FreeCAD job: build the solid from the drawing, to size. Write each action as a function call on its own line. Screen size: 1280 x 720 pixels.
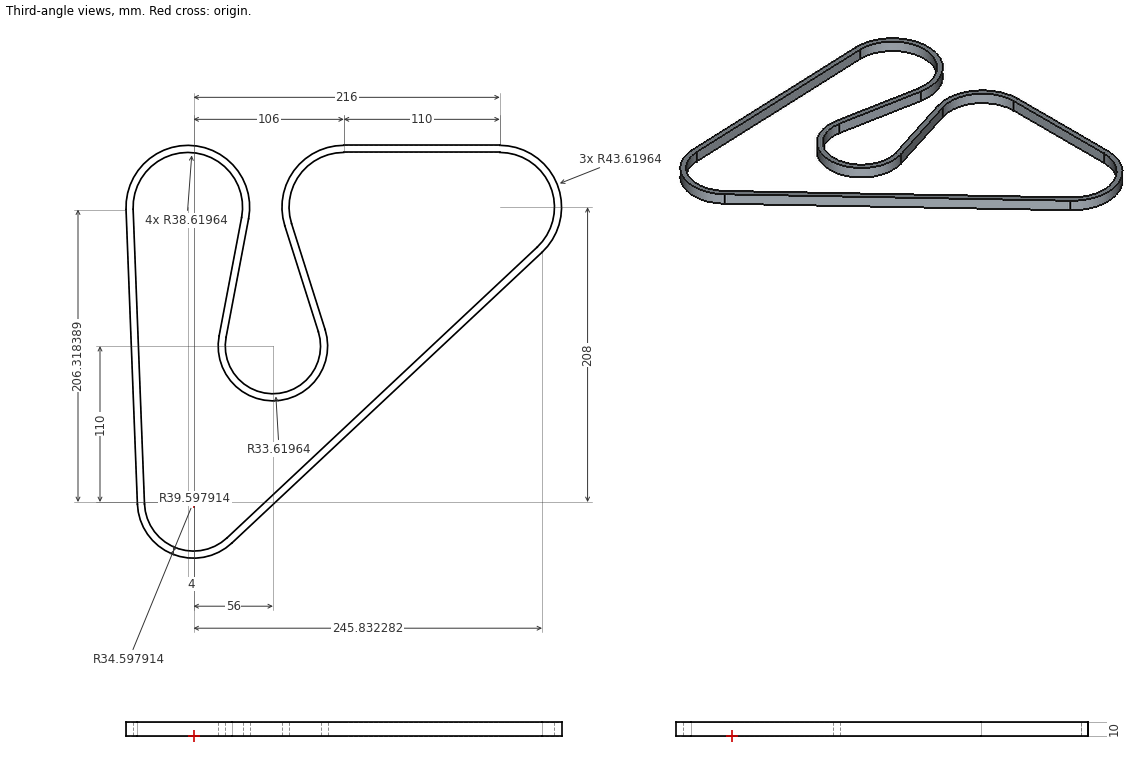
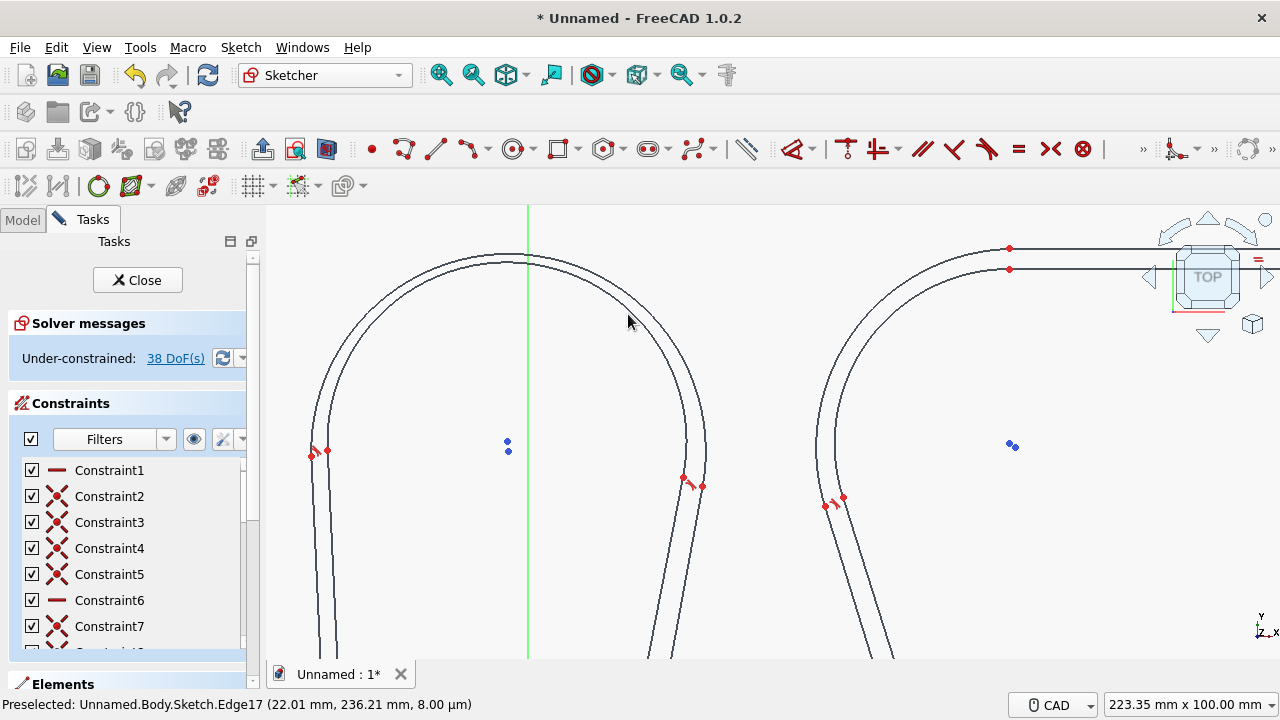
click(661, 591)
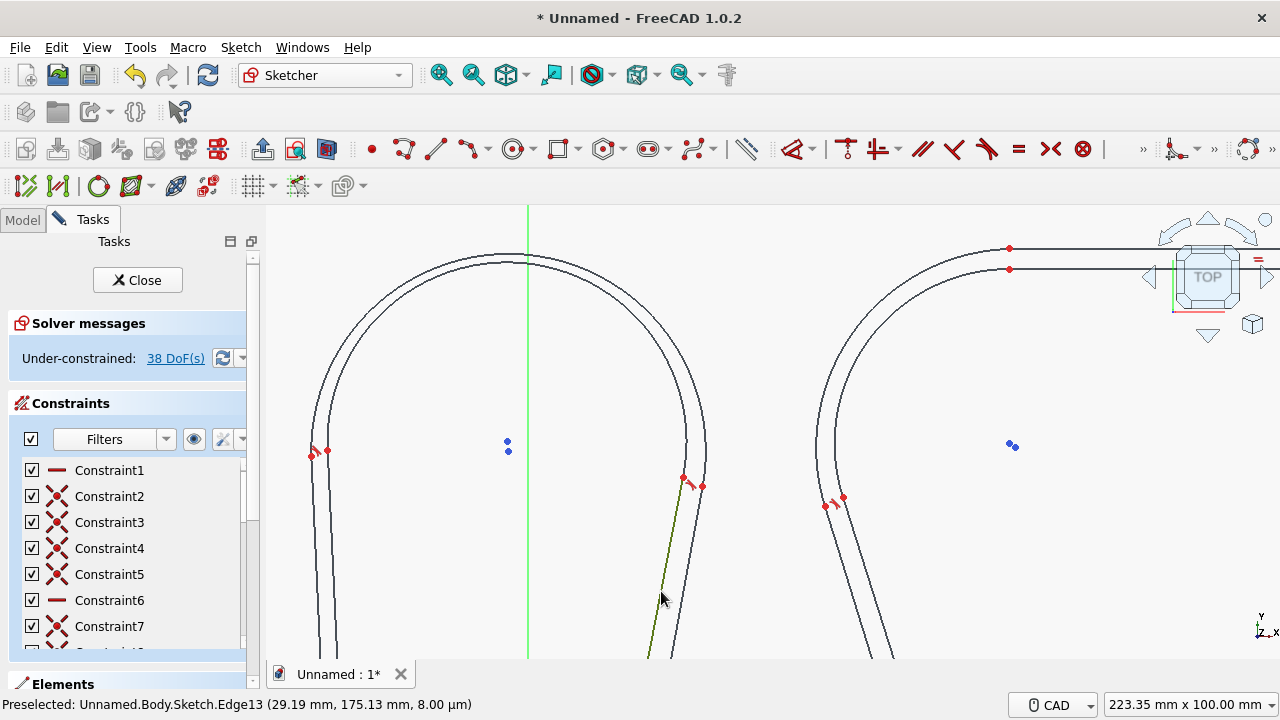
click(630, 311)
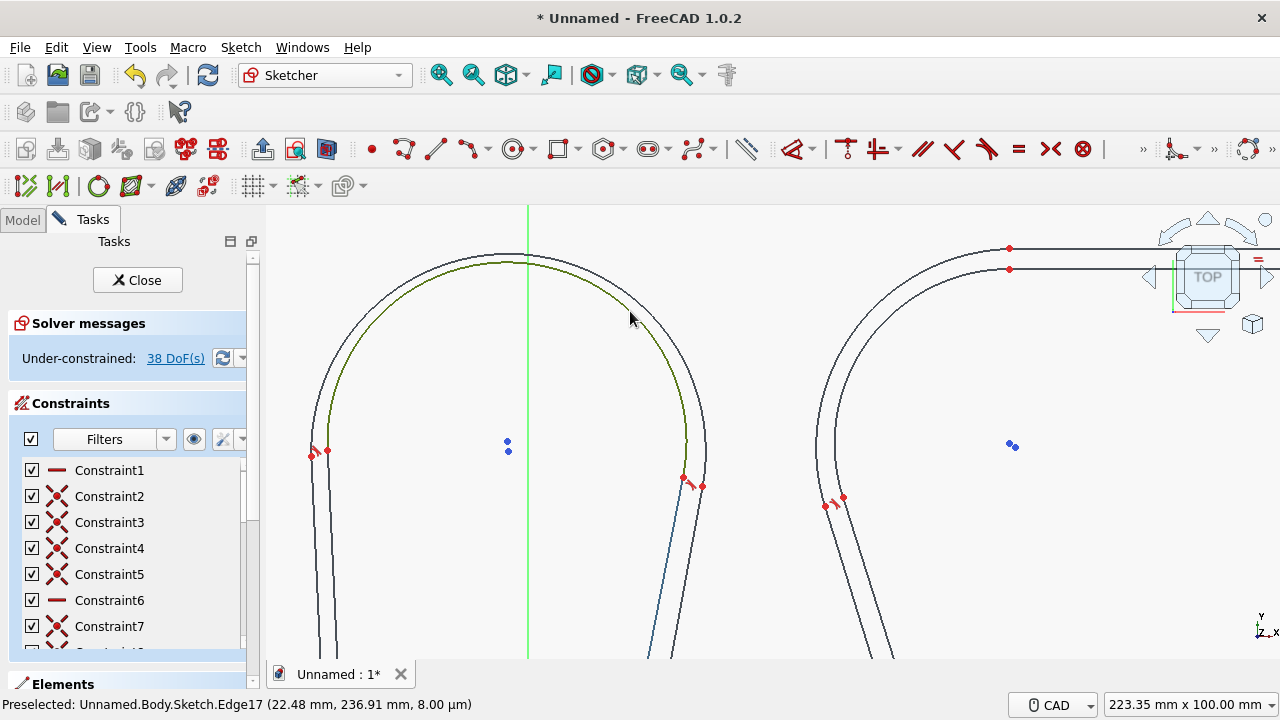
key(t)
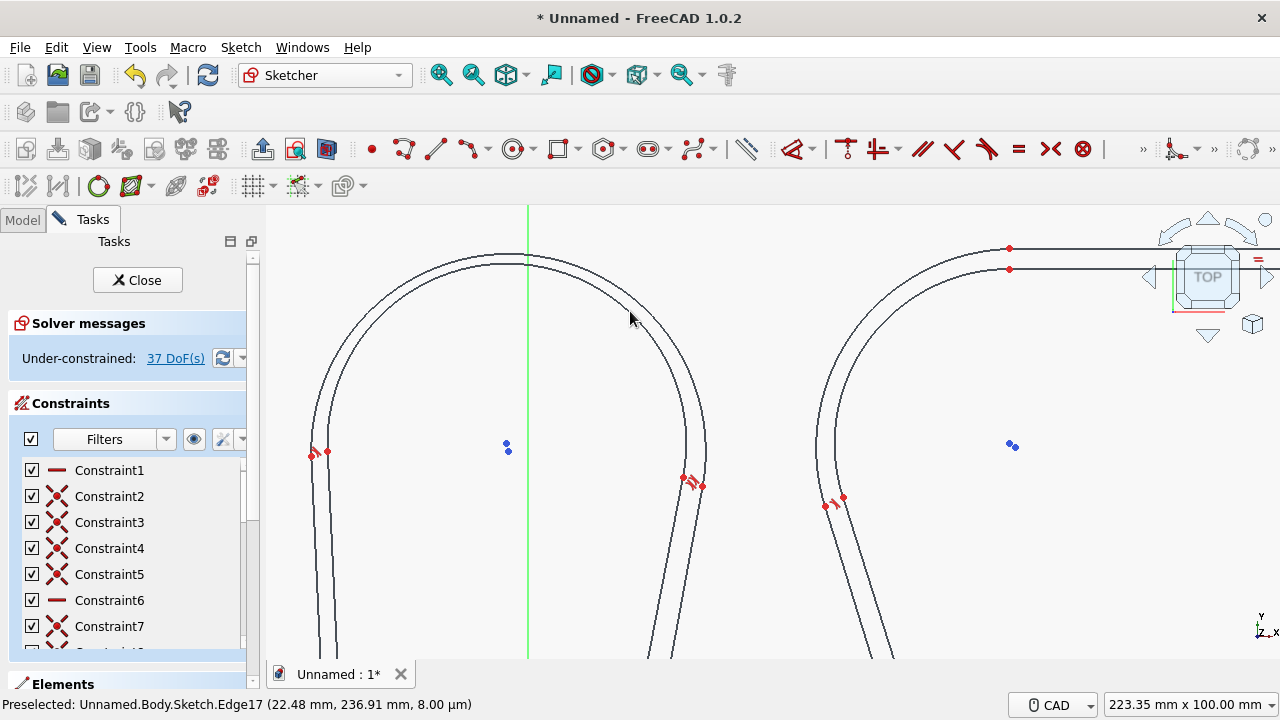
click(661, 591)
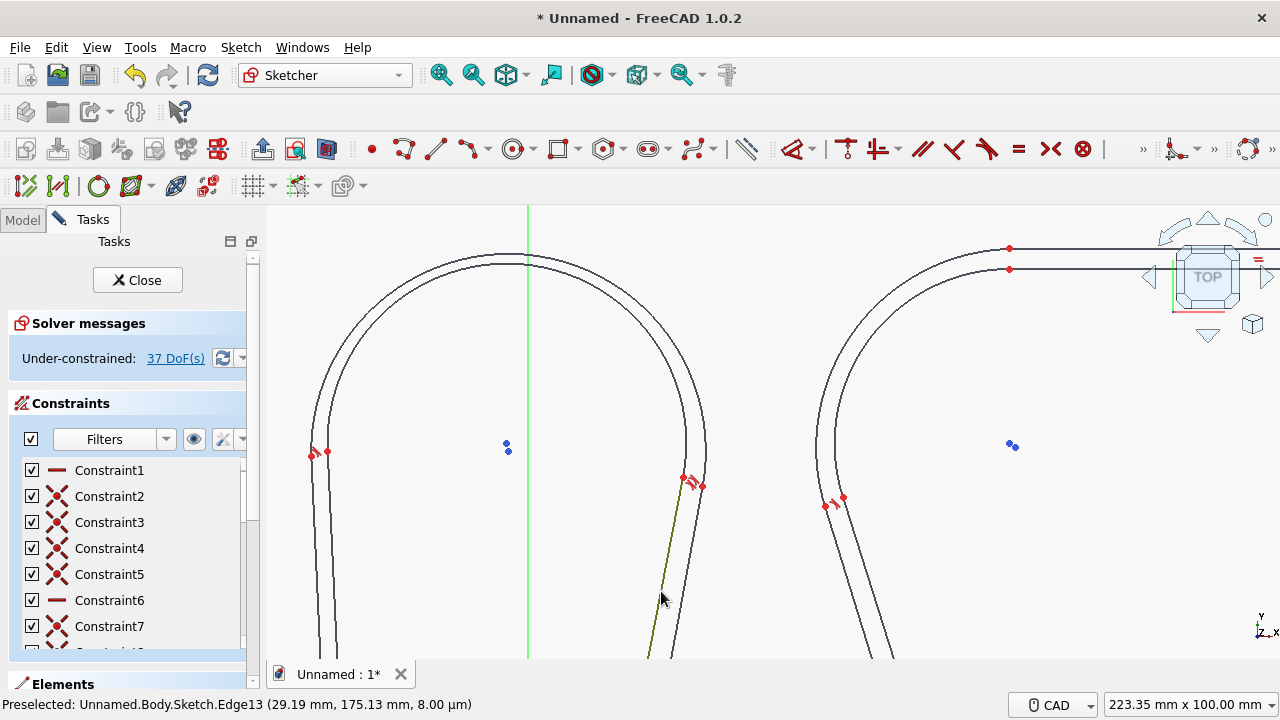
scroll(629, 314, down, 8)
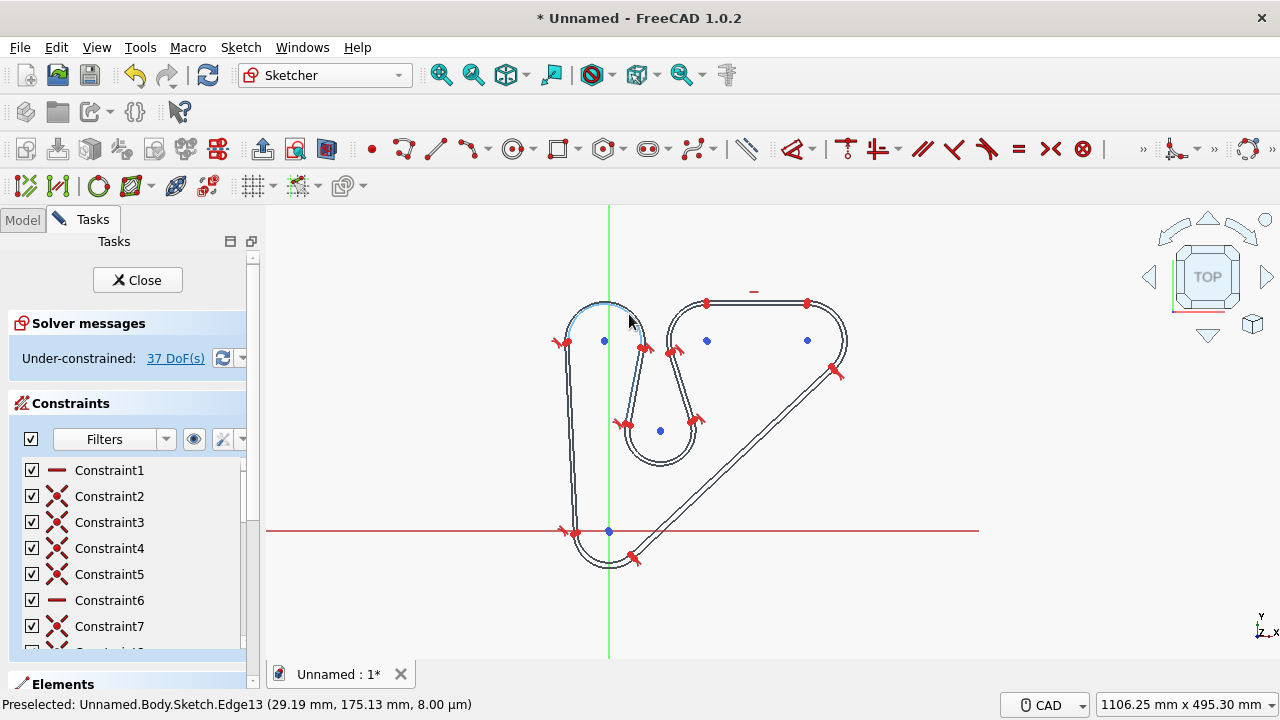
scroll(638, 458, up, 7)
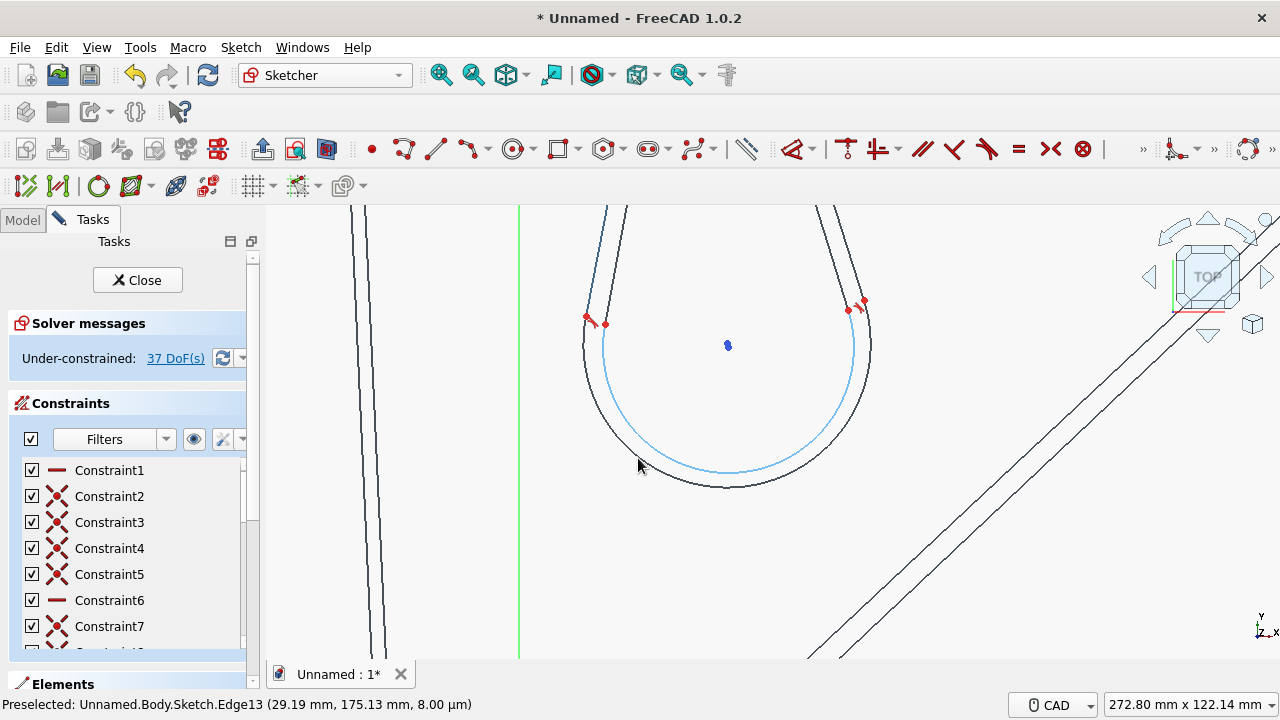
click(638, 457)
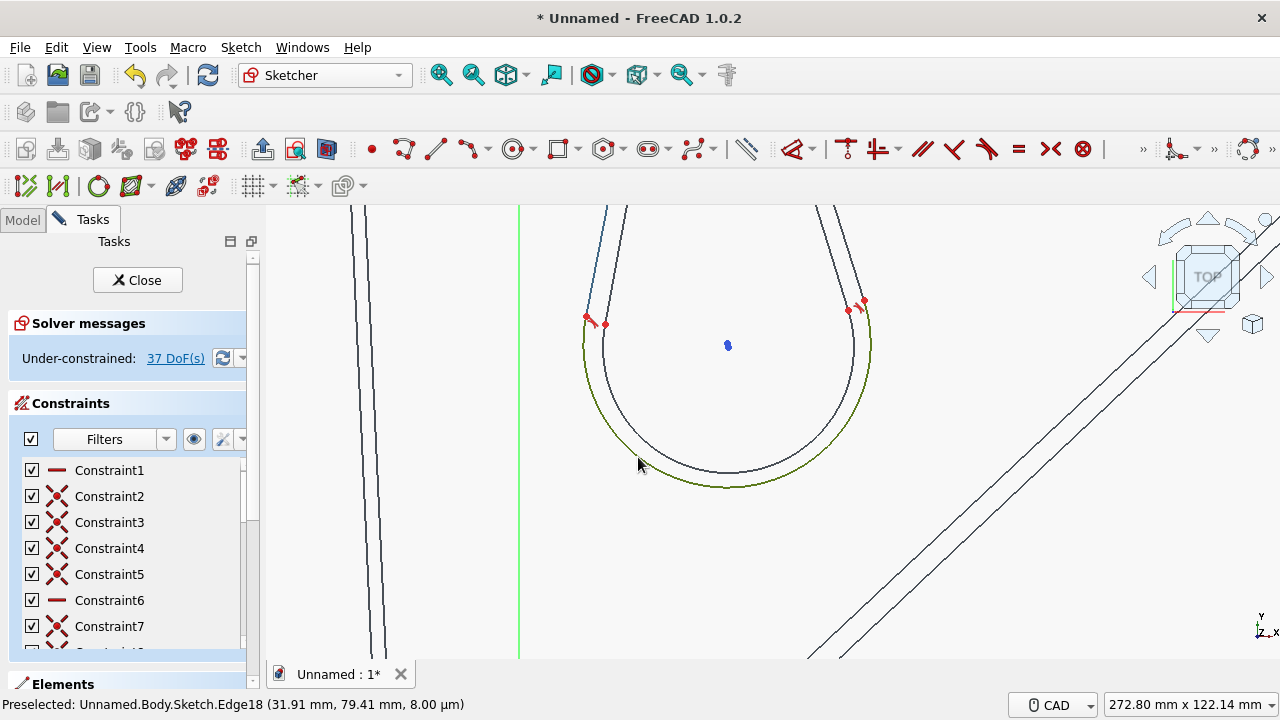
click(988, 150)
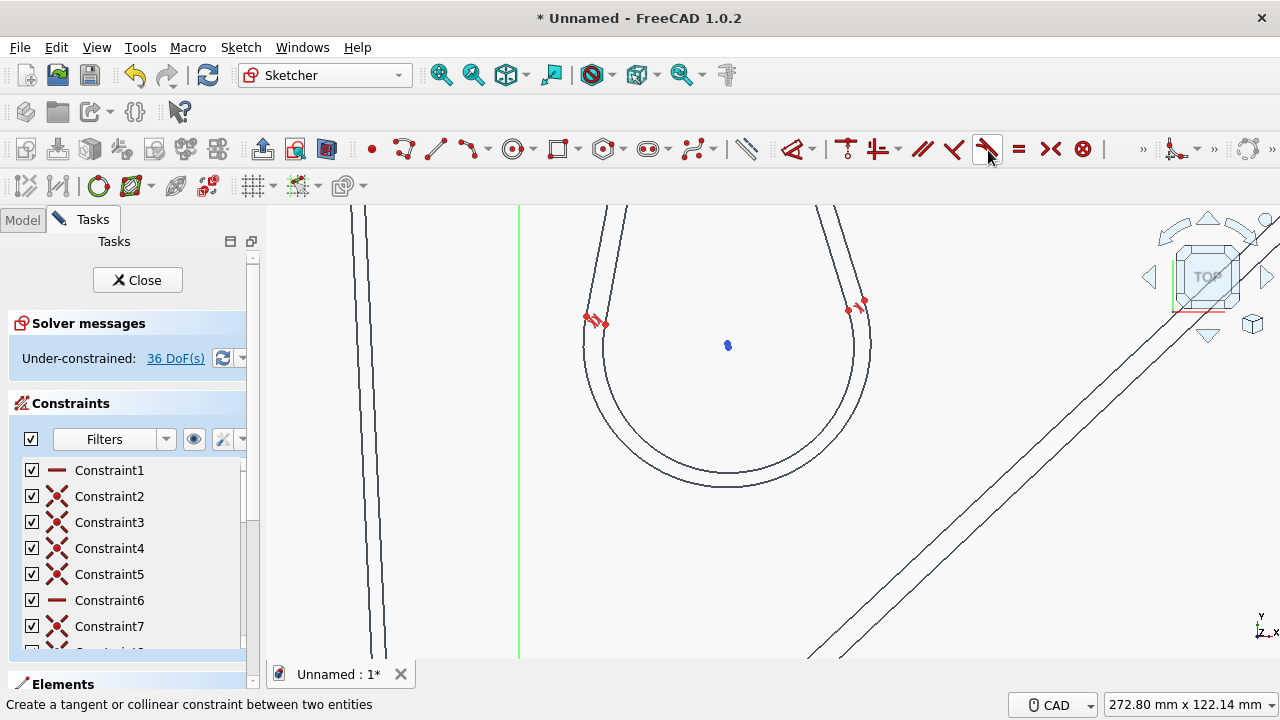
click(847, 245)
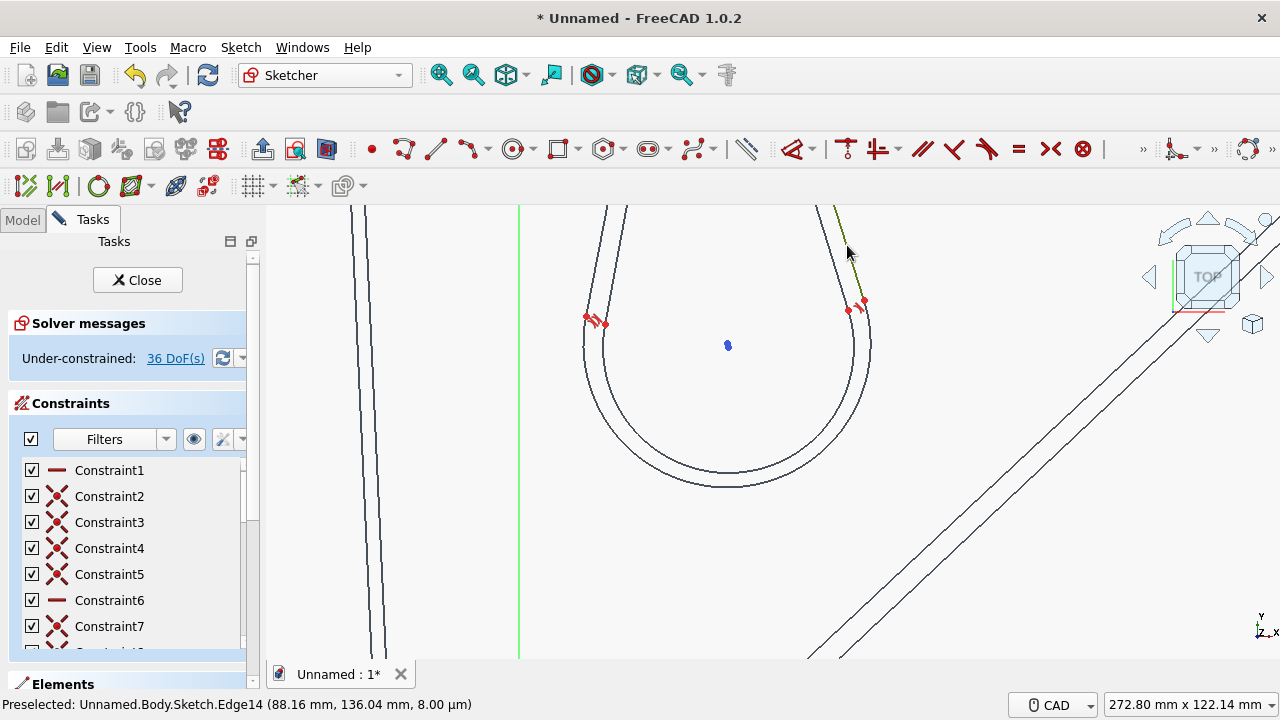
click(638, 456)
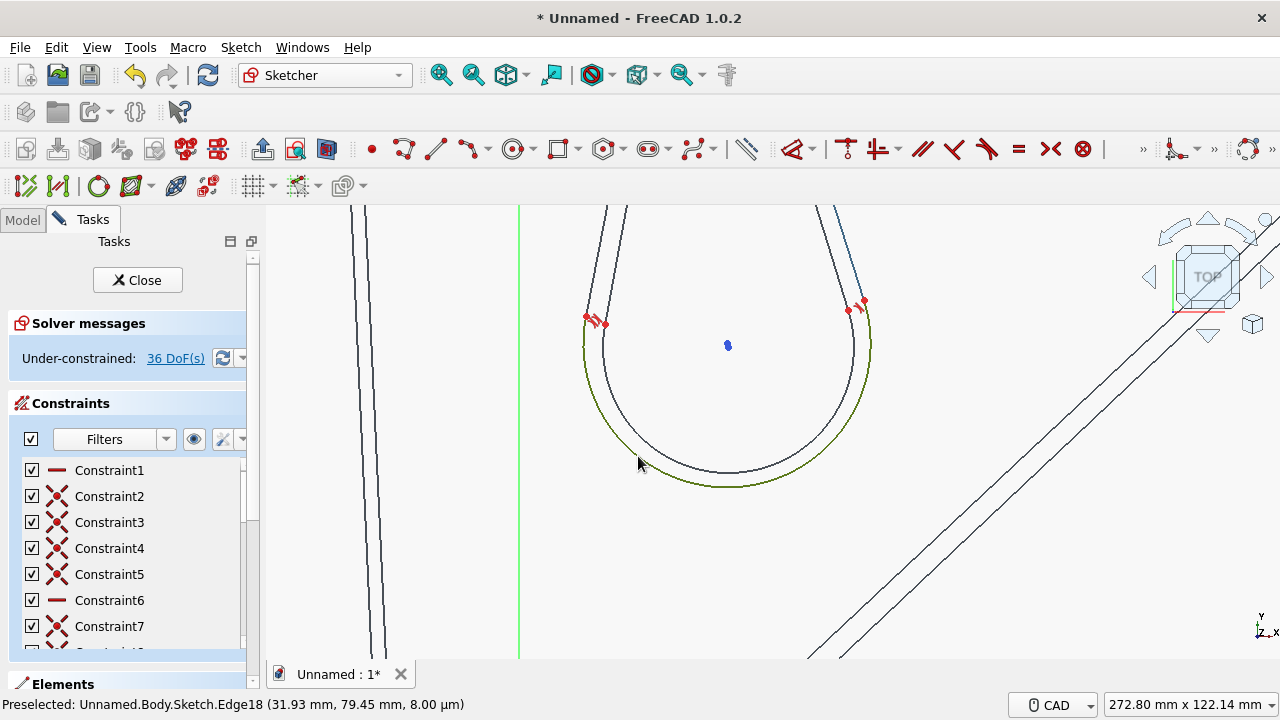
click(988, 150)